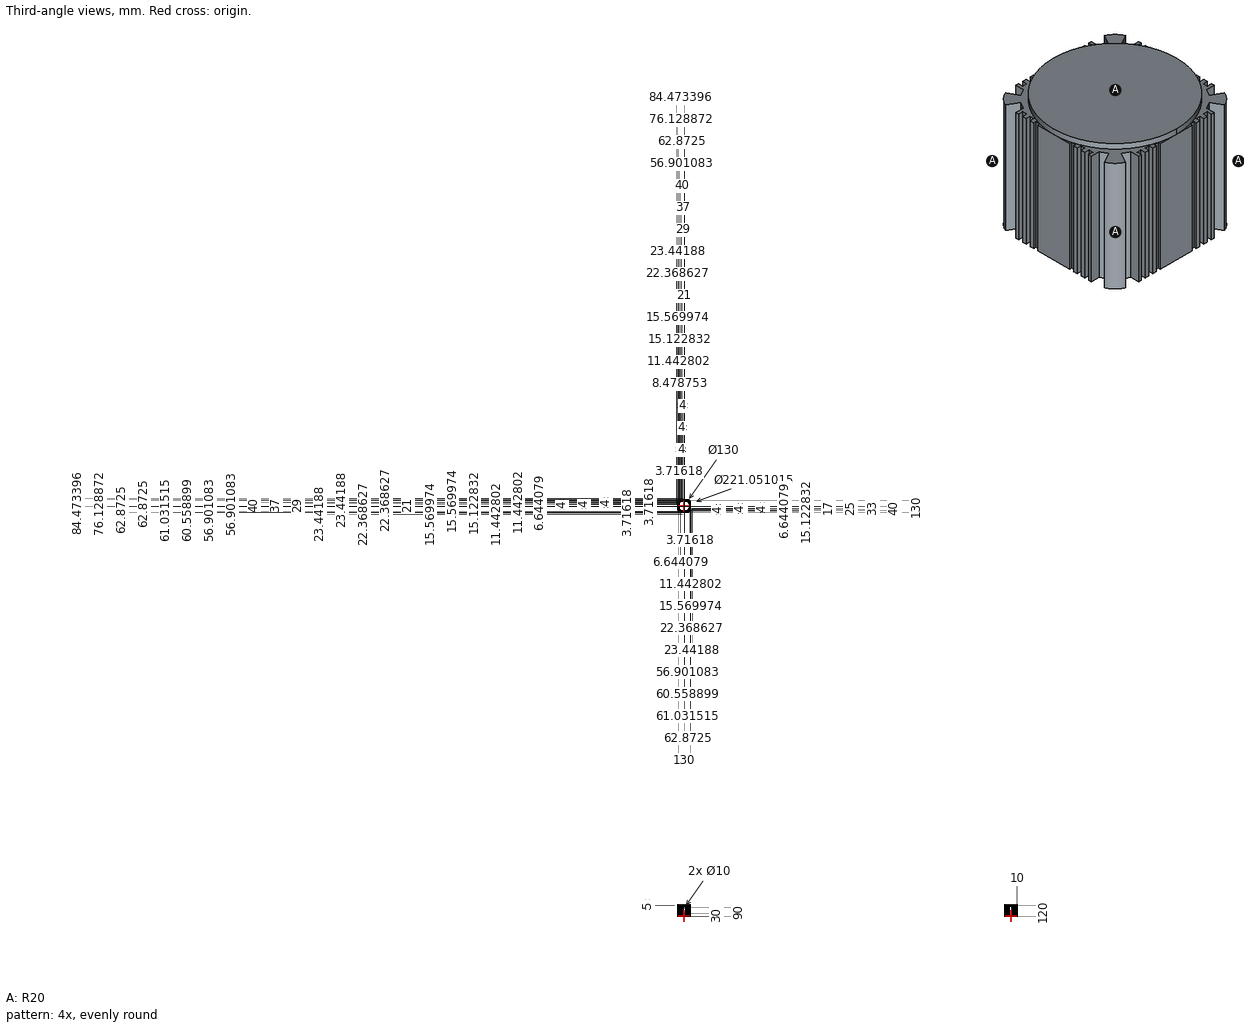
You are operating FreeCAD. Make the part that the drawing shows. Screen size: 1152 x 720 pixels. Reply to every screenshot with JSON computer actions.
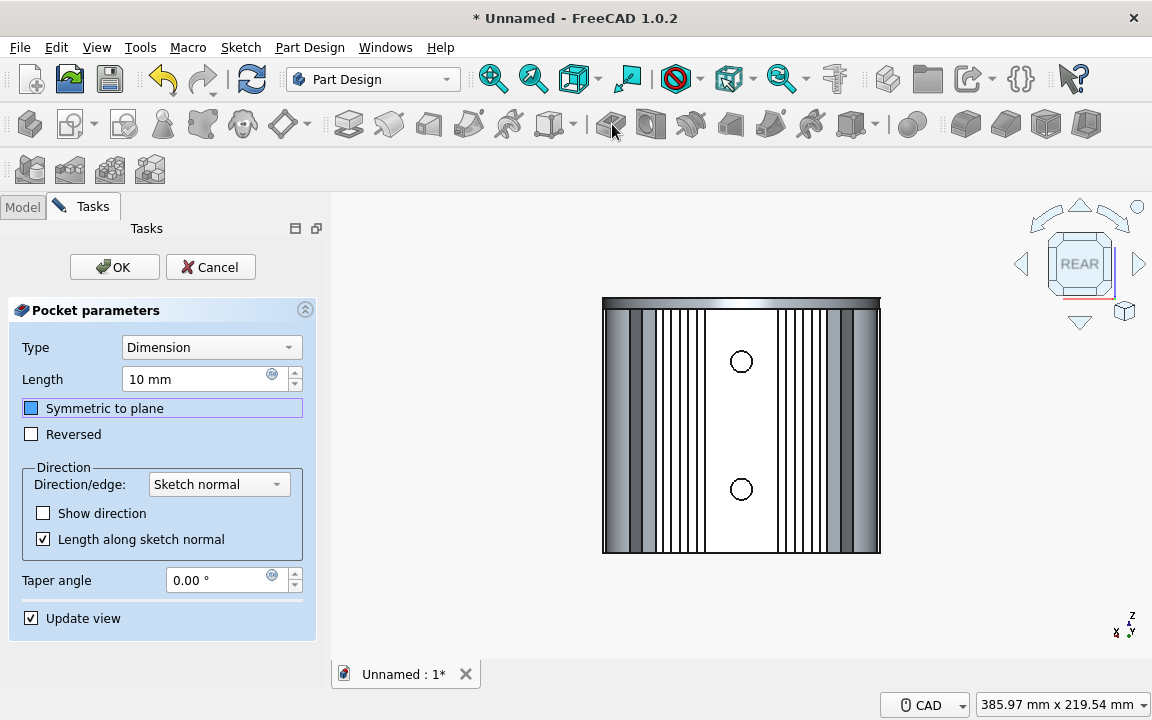
{"action": "left_click", "coordinate": [115, 267]}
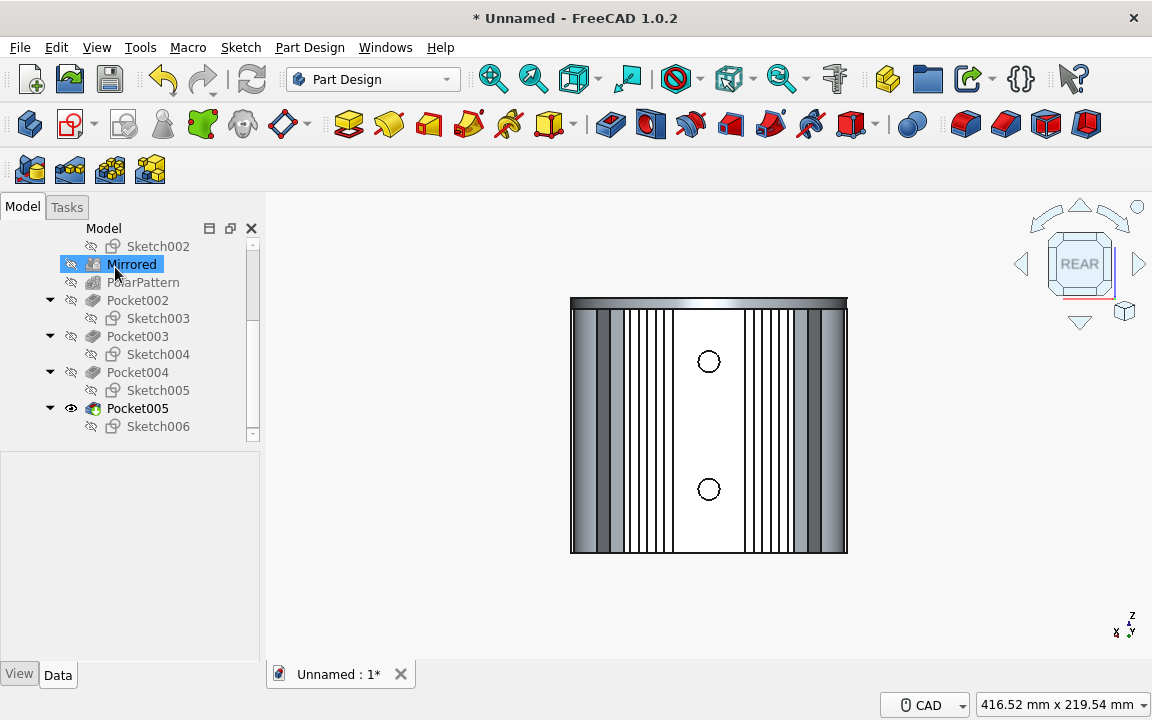
{"action": "key", "text": "0"}